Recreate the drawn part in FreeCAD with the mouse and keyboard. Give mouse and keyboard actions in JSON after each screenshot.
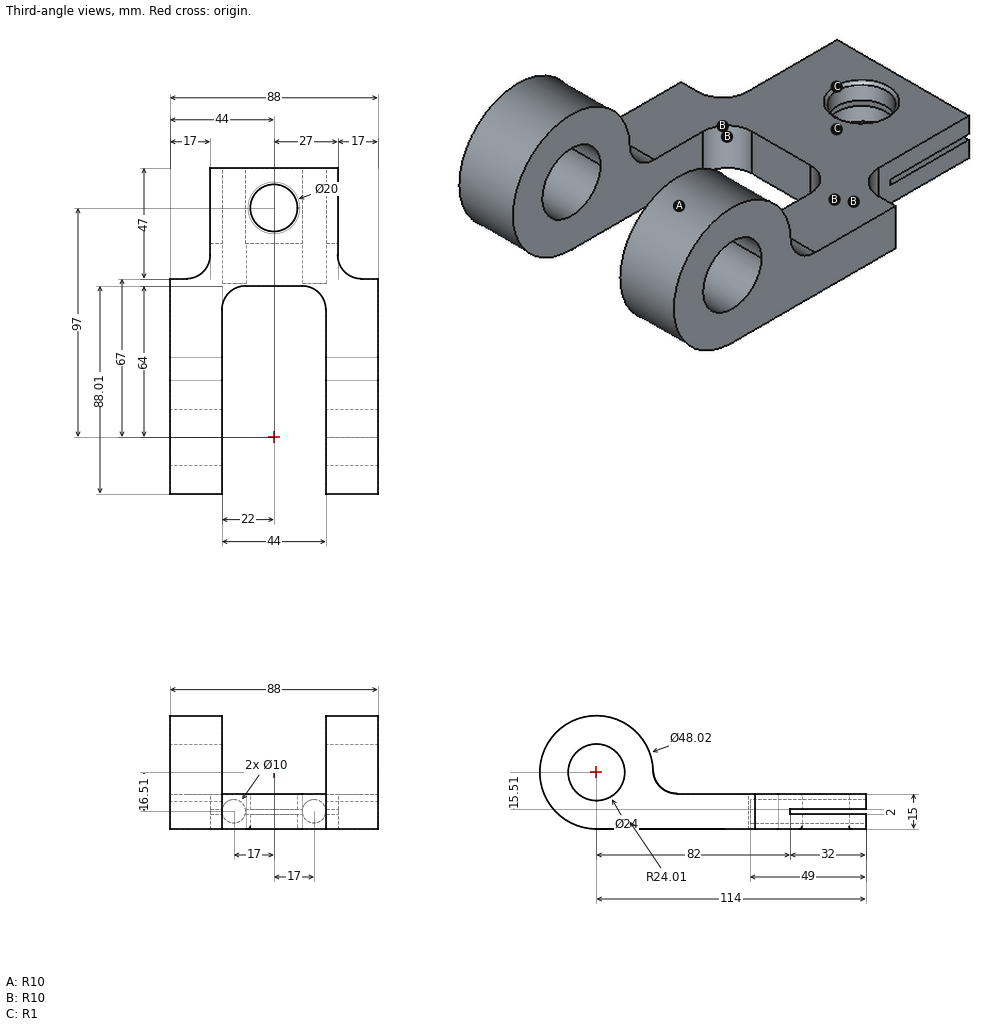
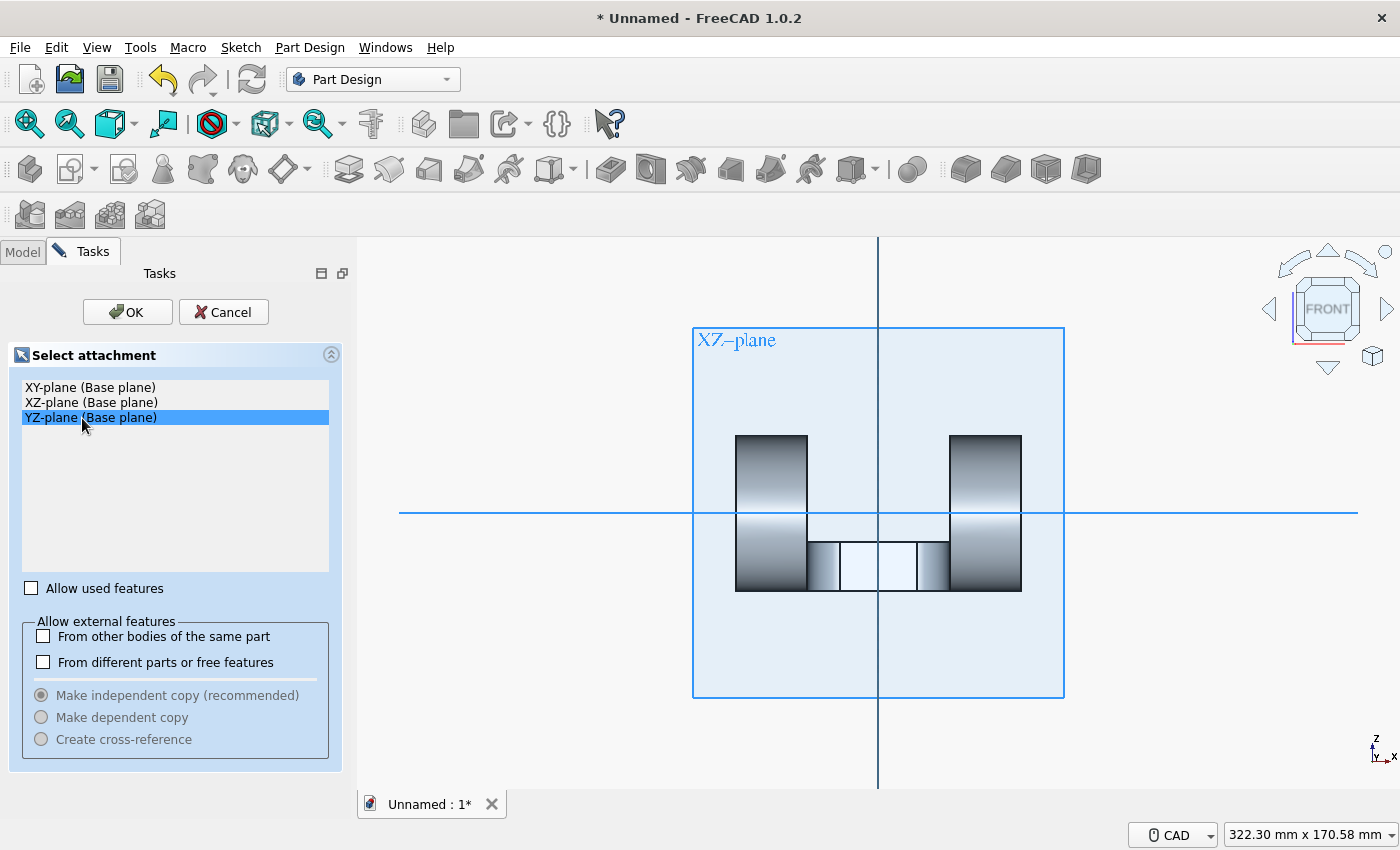
{"action": "left_click", "coordinate": [128, 312]}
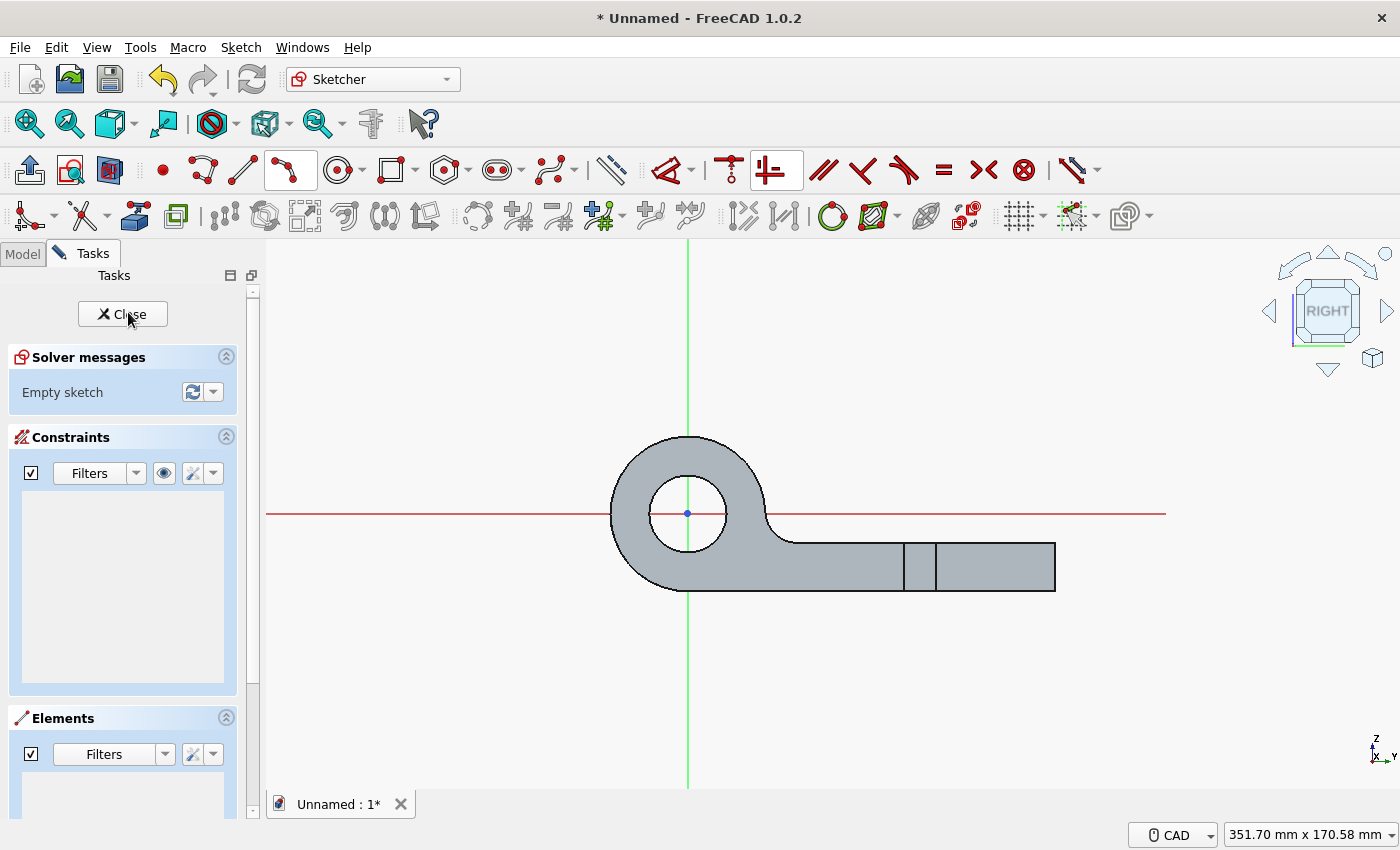
{"action": "left_click", "coordinate": [110, 170]}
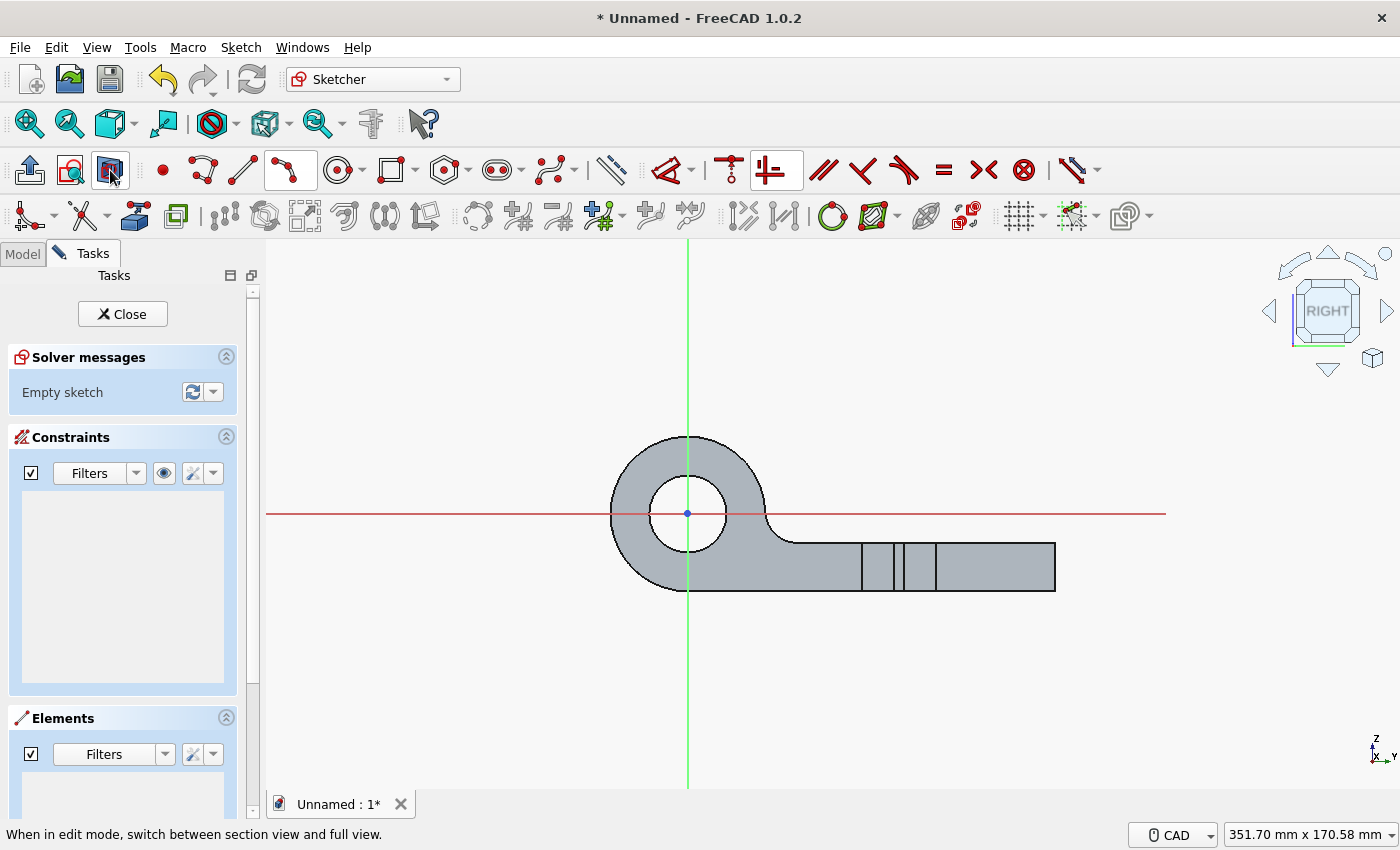
{"action": "scroll", "coordinate": [1051, 578], "scroll_direction": "up", "scroll_amount": 9}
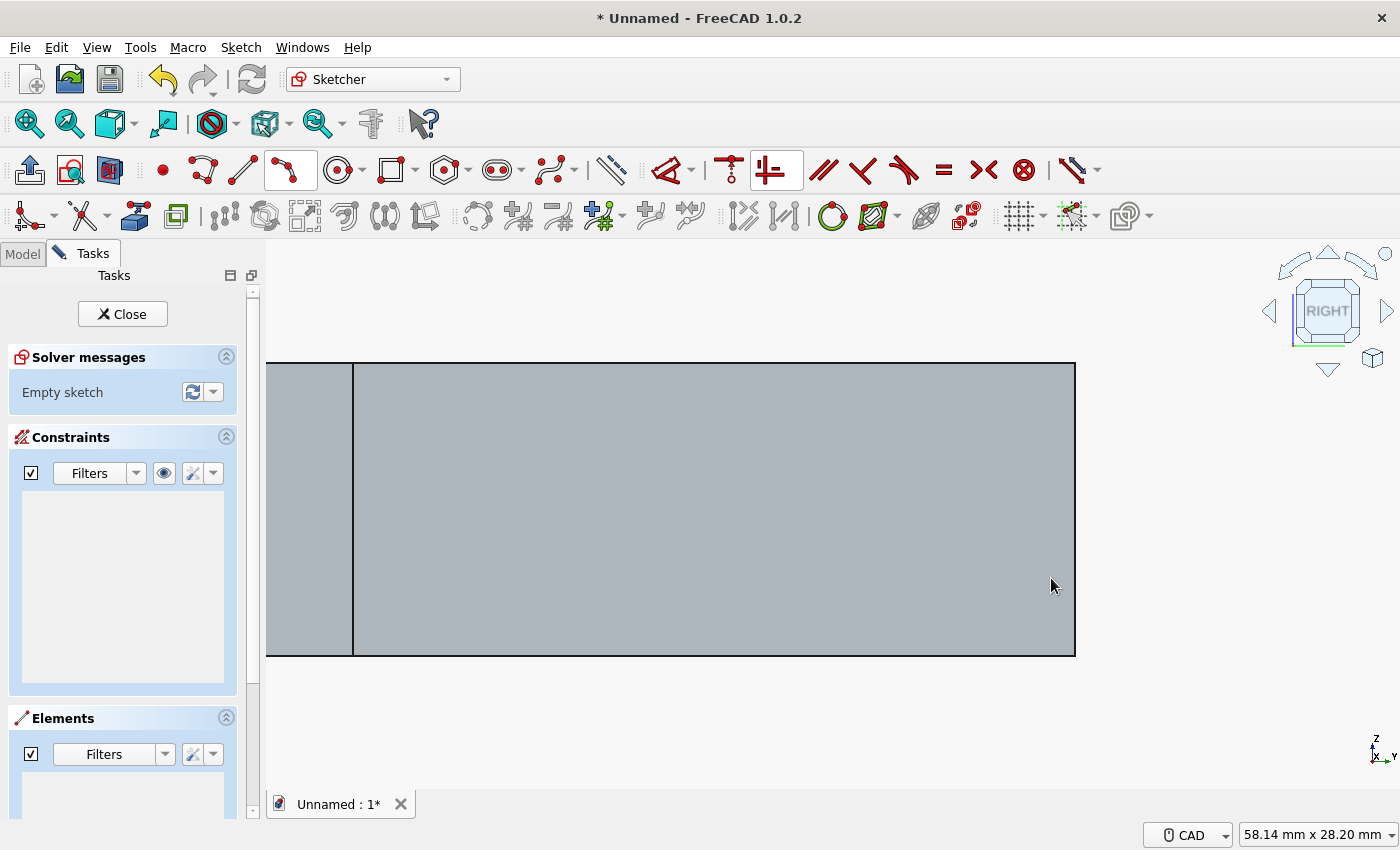
{"action": "left_click", "coordinate": [392, 170]}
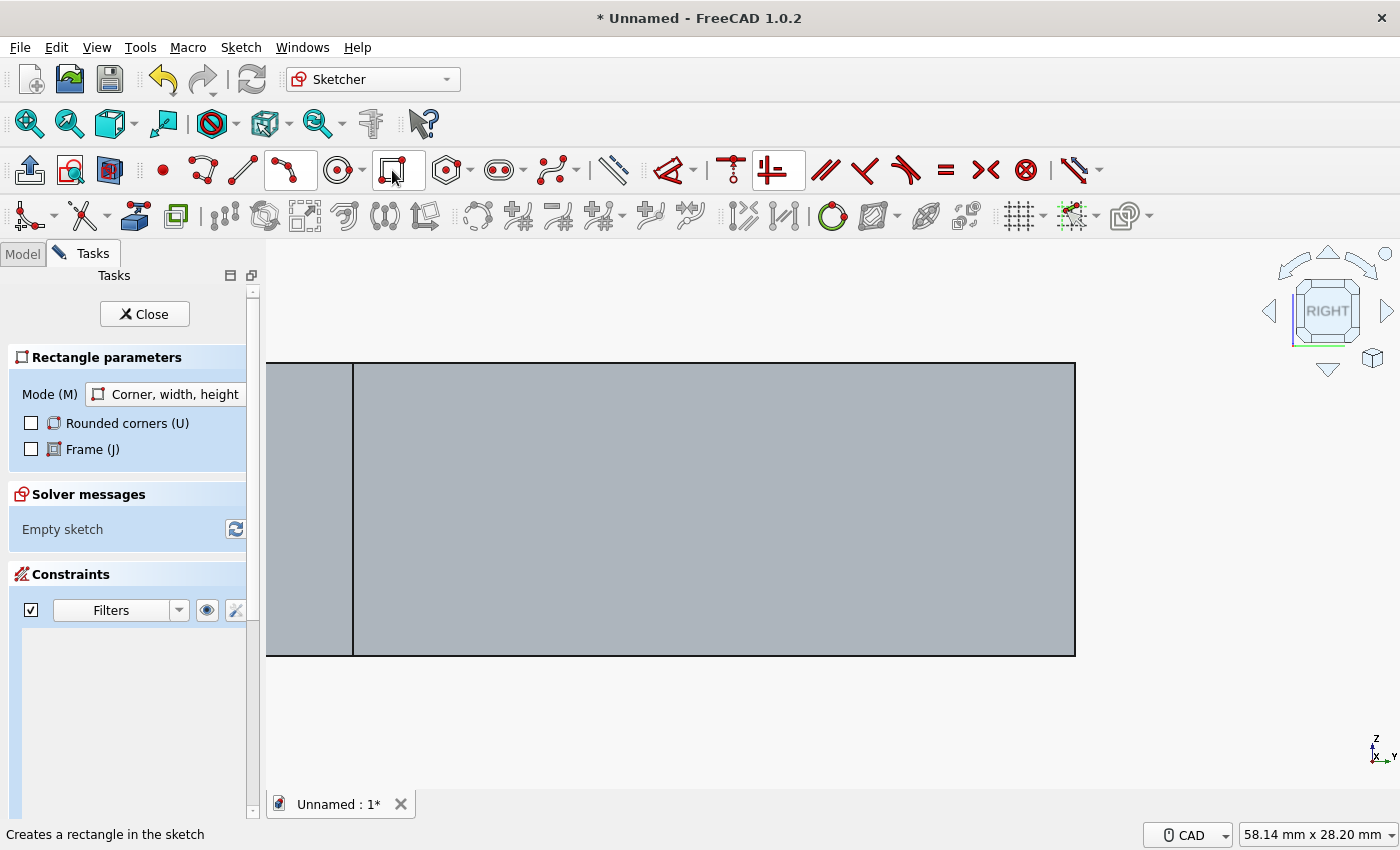
{"action": "left_click", "coordinate": [451, 490]}
{"action": "left_click", "coordinate": [1075, 529]}
{"action": "key", "text": "Escape"}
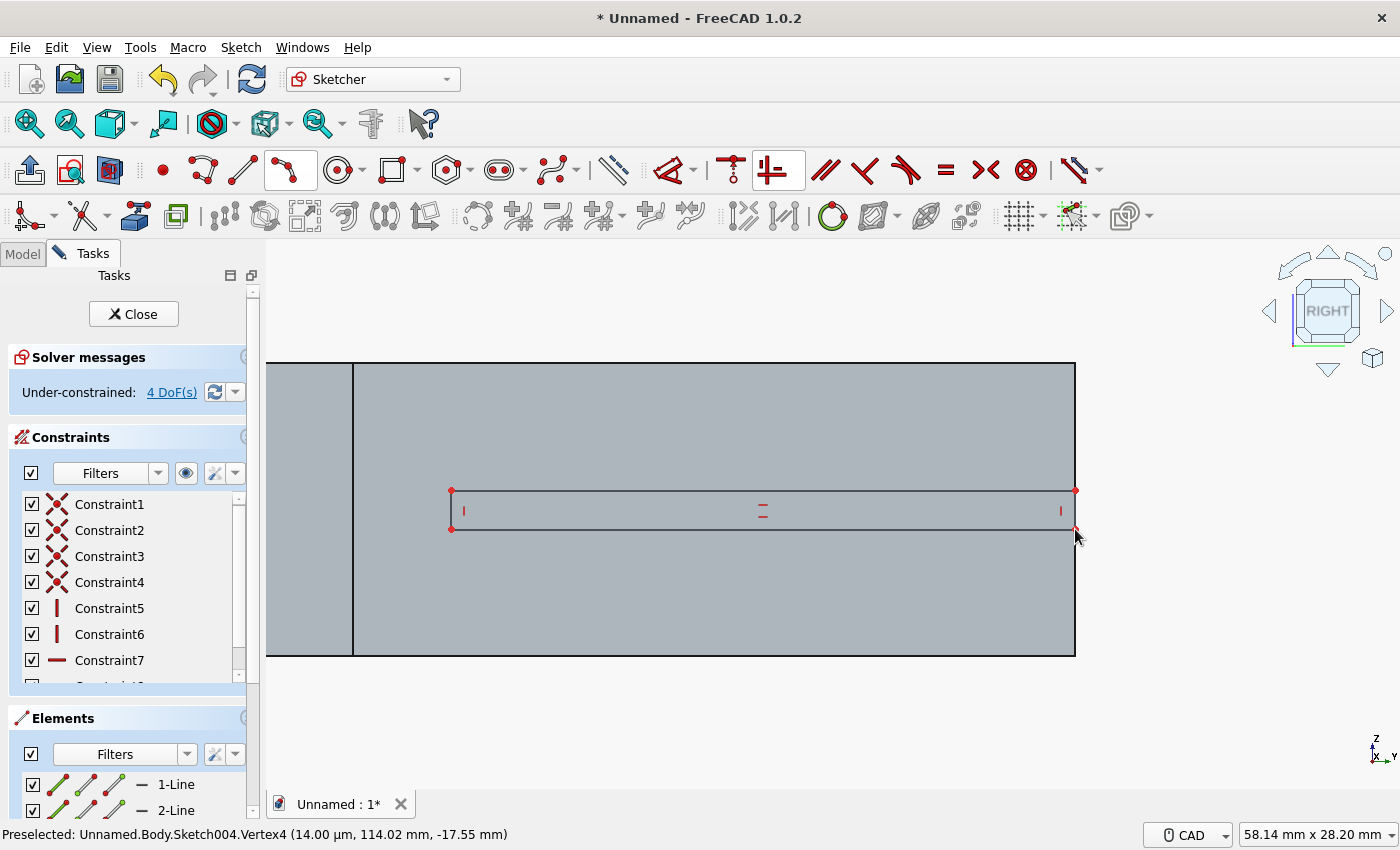
{"action": "left_click", "coordinate": [668, 170]}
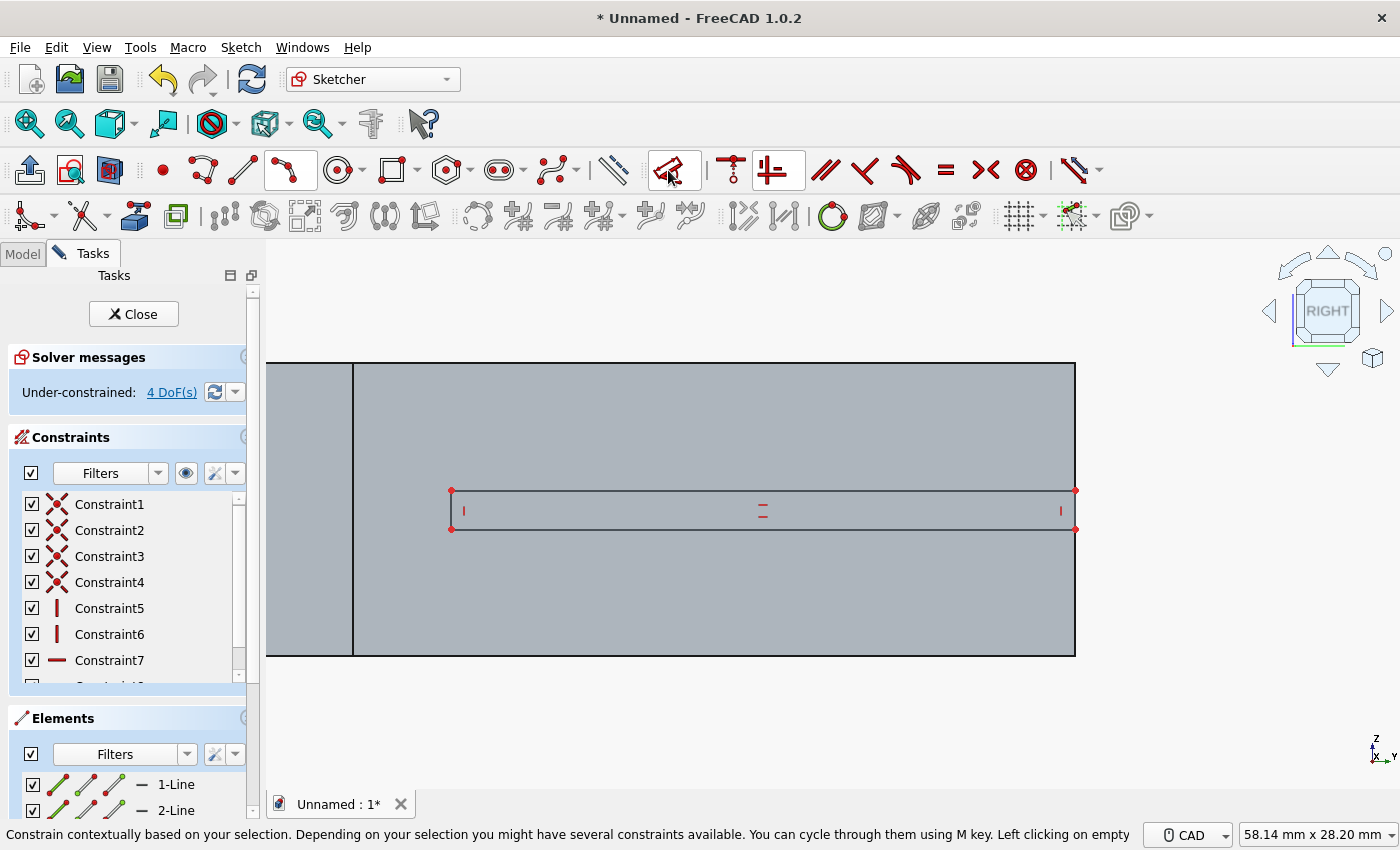
{"action": "left_click", "coordinate": [451, 503]}
{"action": "left_click", "coordinate": [417, 510]}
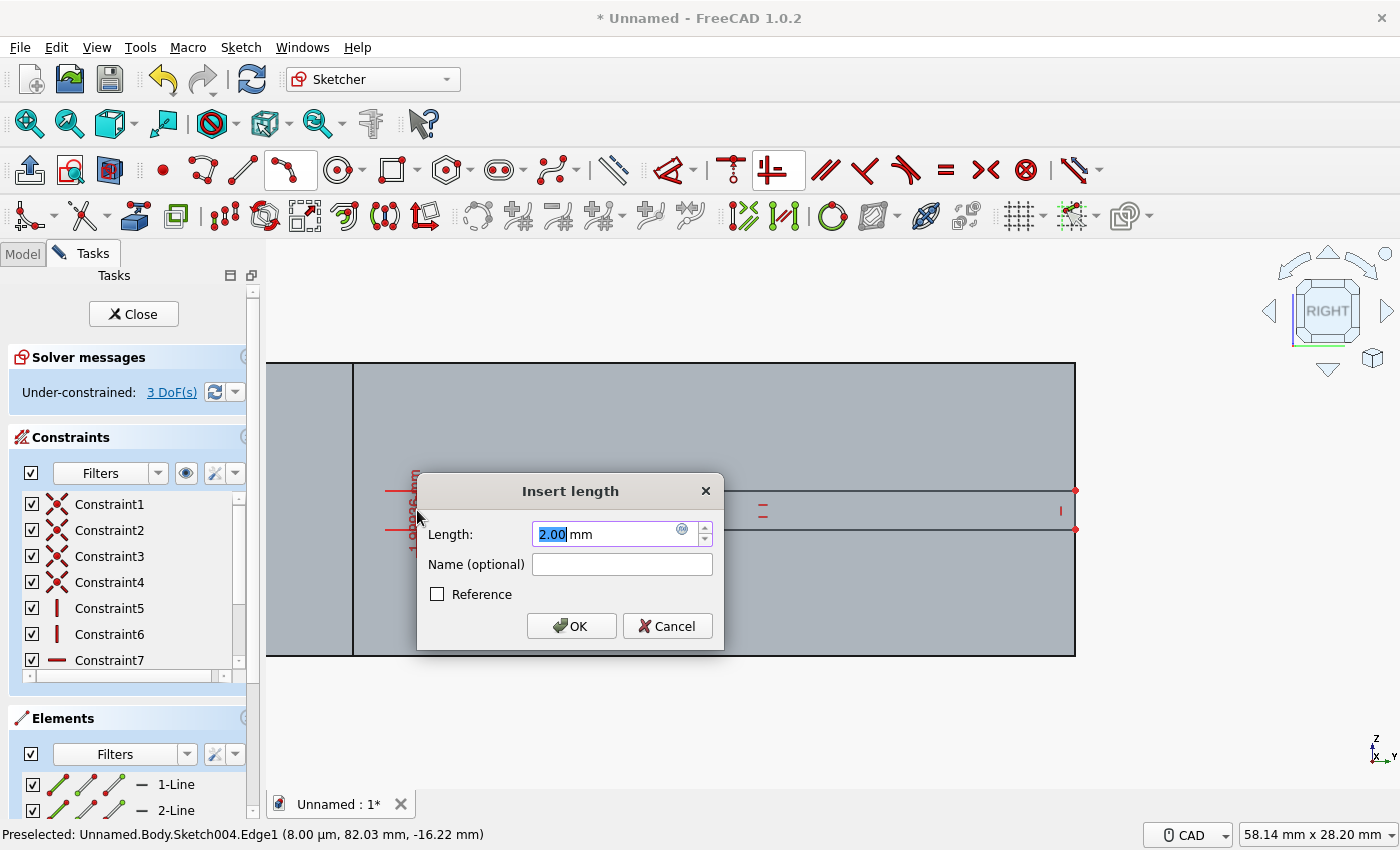
{"action": "type", "text": "2"}
{"action": "key", "text": "Return"}